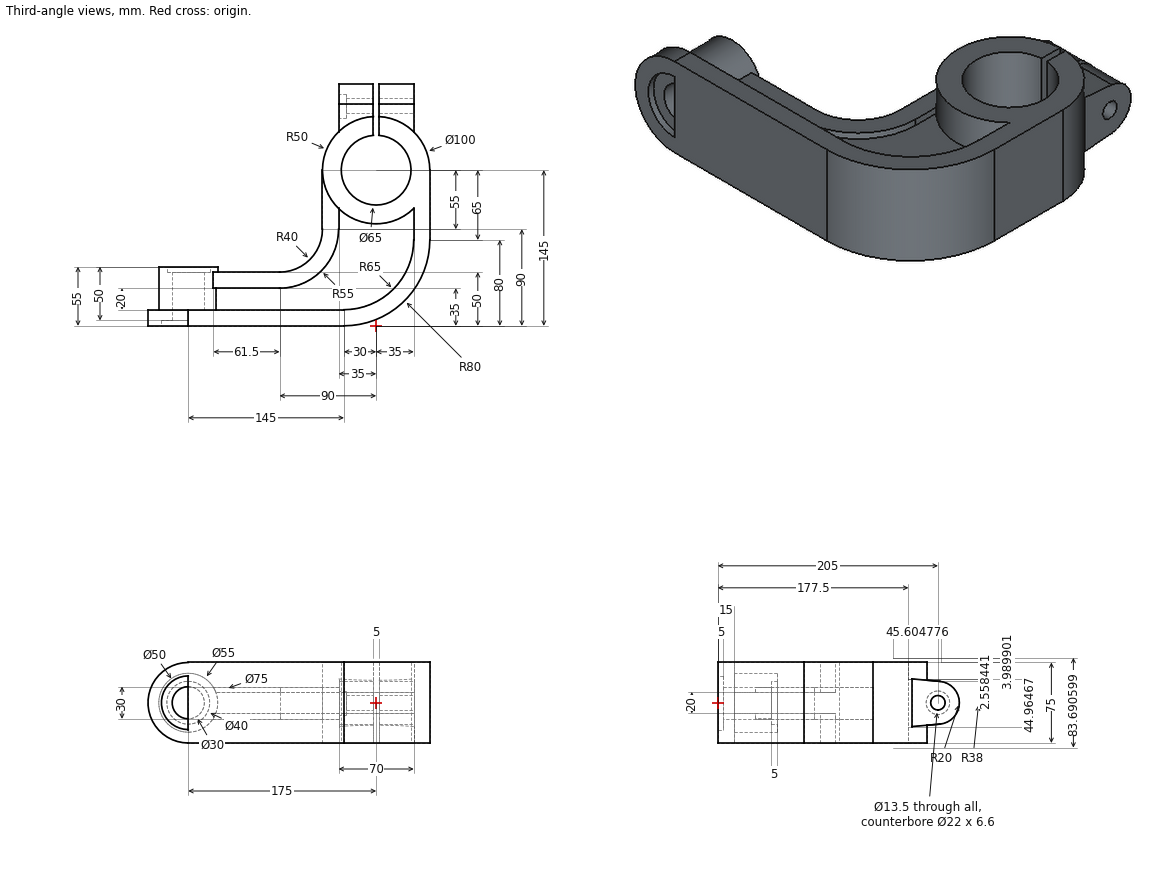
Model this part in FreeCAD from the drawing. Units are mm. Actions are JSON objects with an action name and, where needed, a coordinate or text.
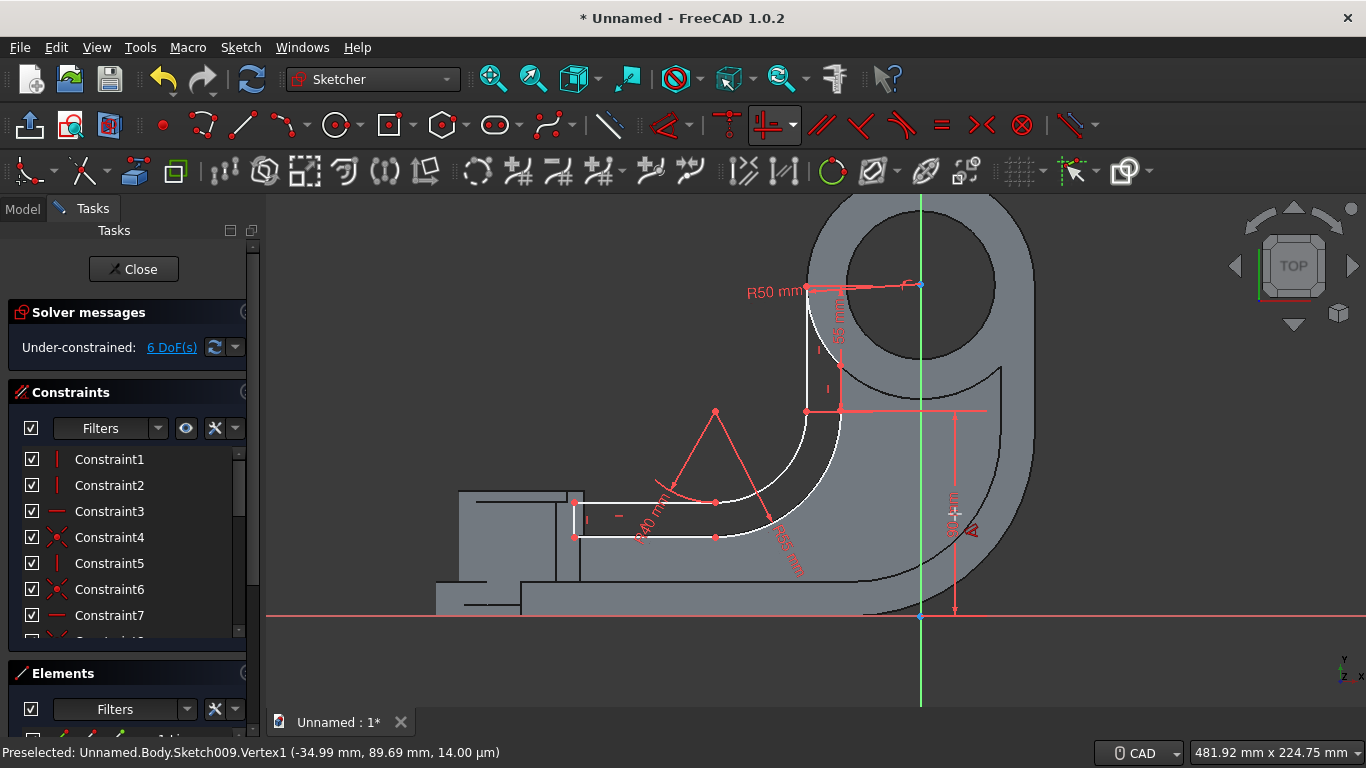
{"action": "left_click", "coordinate": [807, 412]}
{"action": "left_click", "coordinate": [955, 467]}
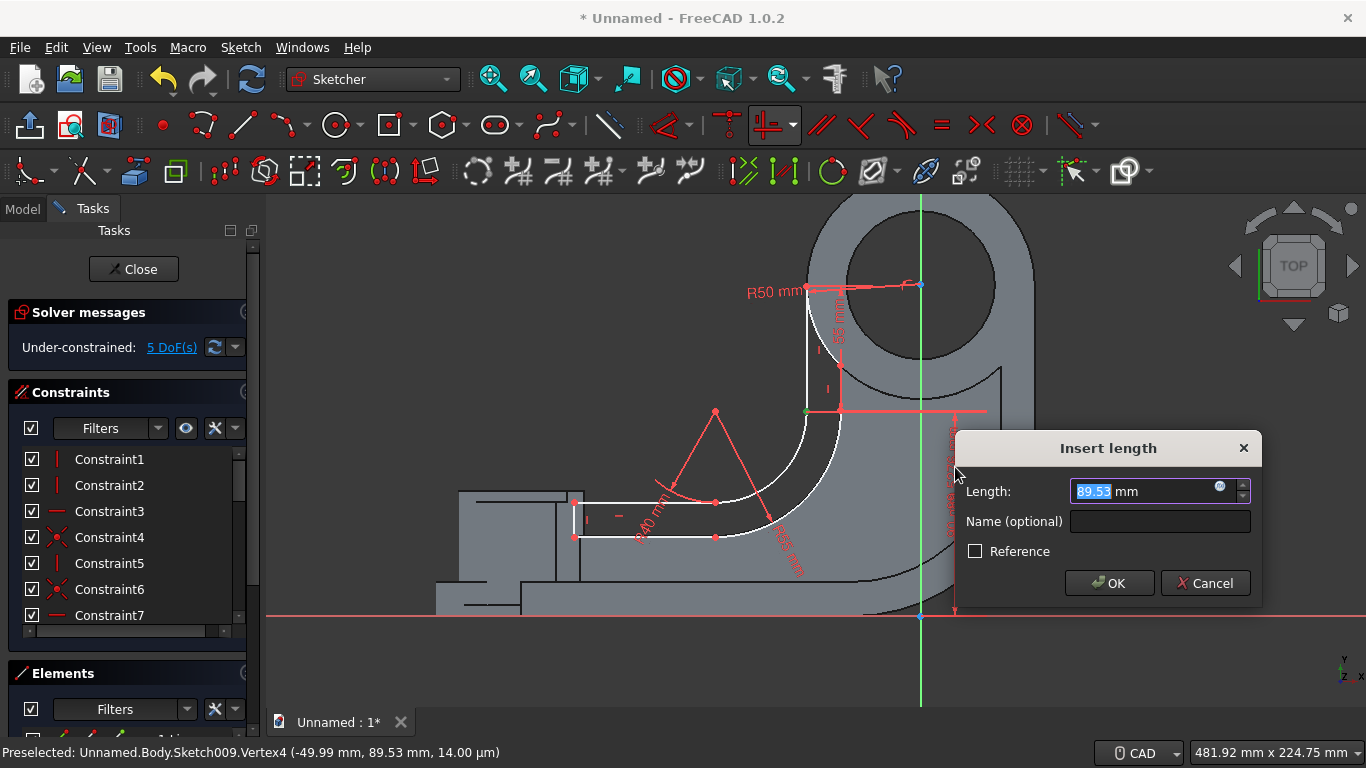
{"action": "type", "text": "90"}
{"action": "key", "text": "Return"}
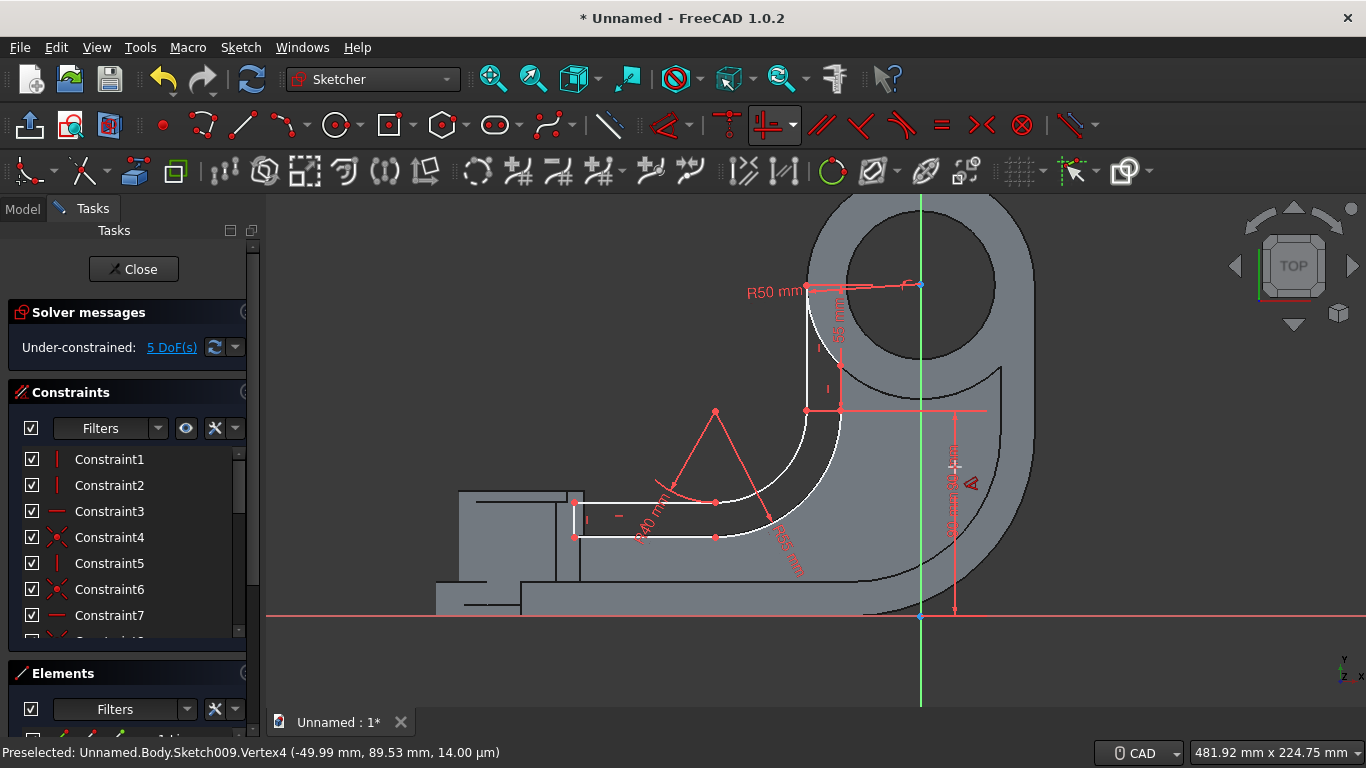
{"action": "left_click", "coordinate": [715, 503]}
{"action": "left_click", "coordinate": [818, 650]}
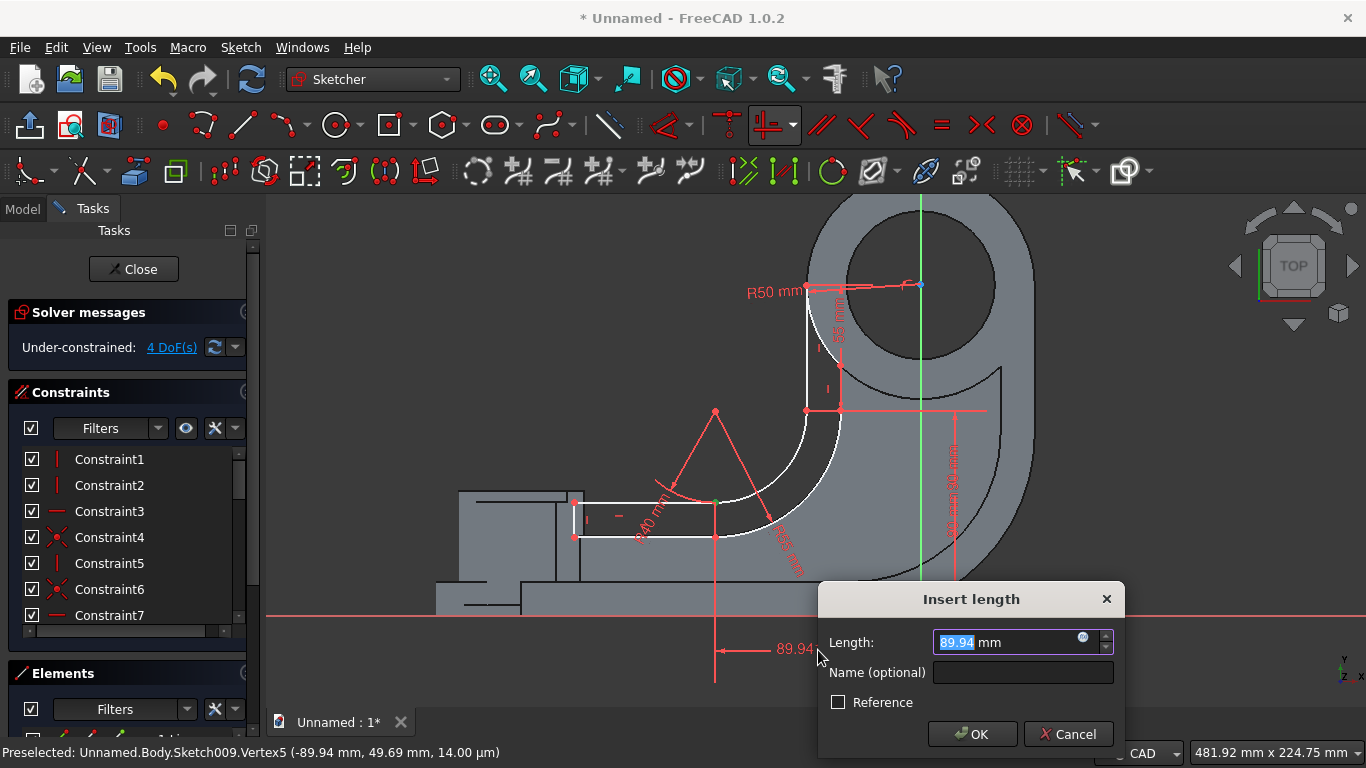
{"action": "type", "text": "90"}
{"action": "key", "text": "Return"}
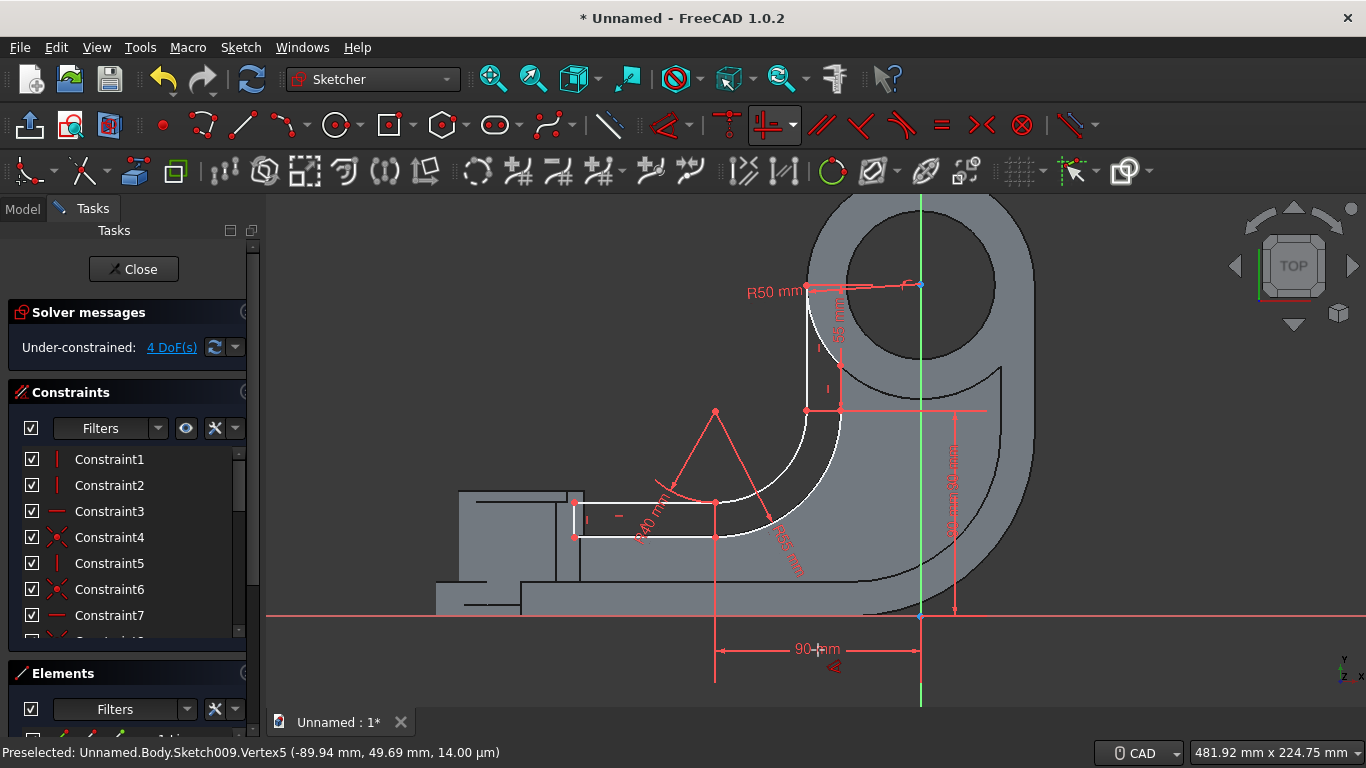
{"action": "left_click", "coordinate": [715, 503]}
{"action": "left_click", "coordinate": [955, 559]}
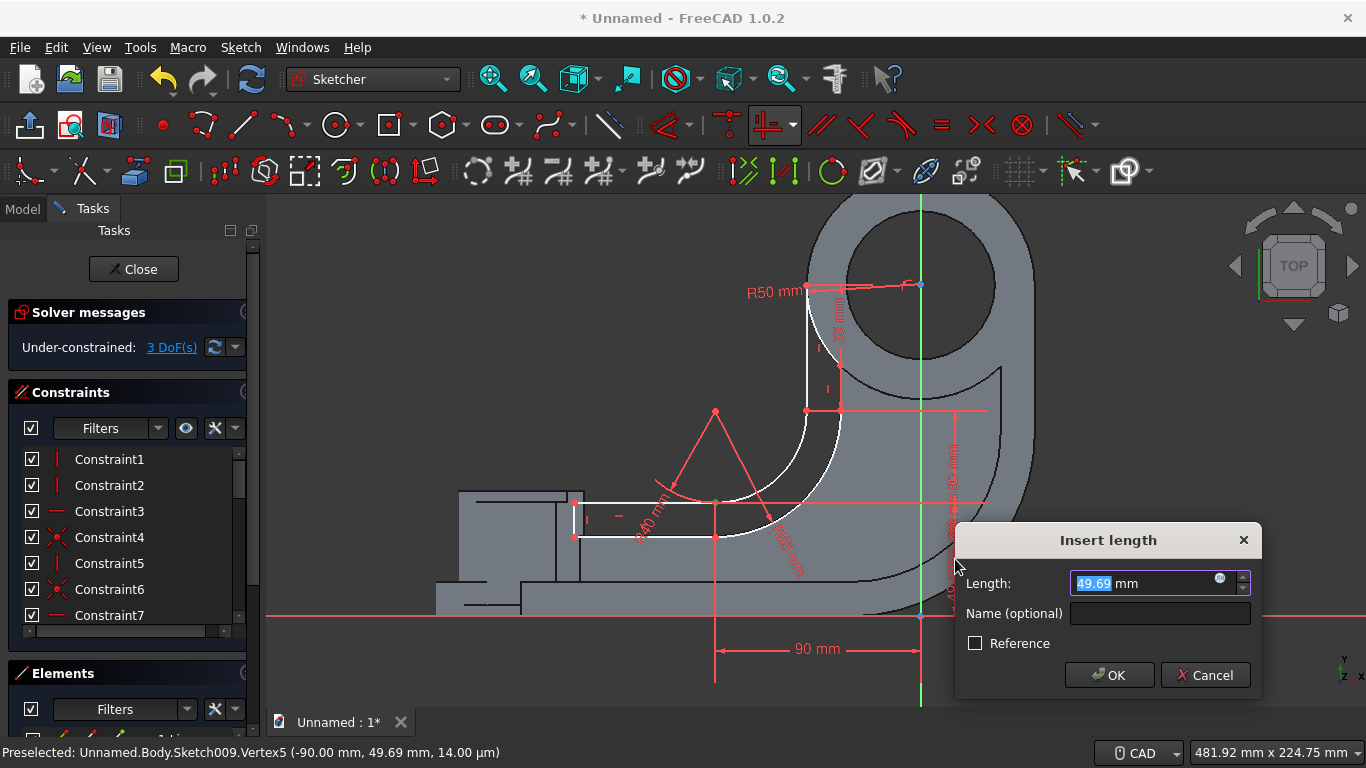
{"action": "type", "text": "50"}
{"action": "key", "text": "Return"}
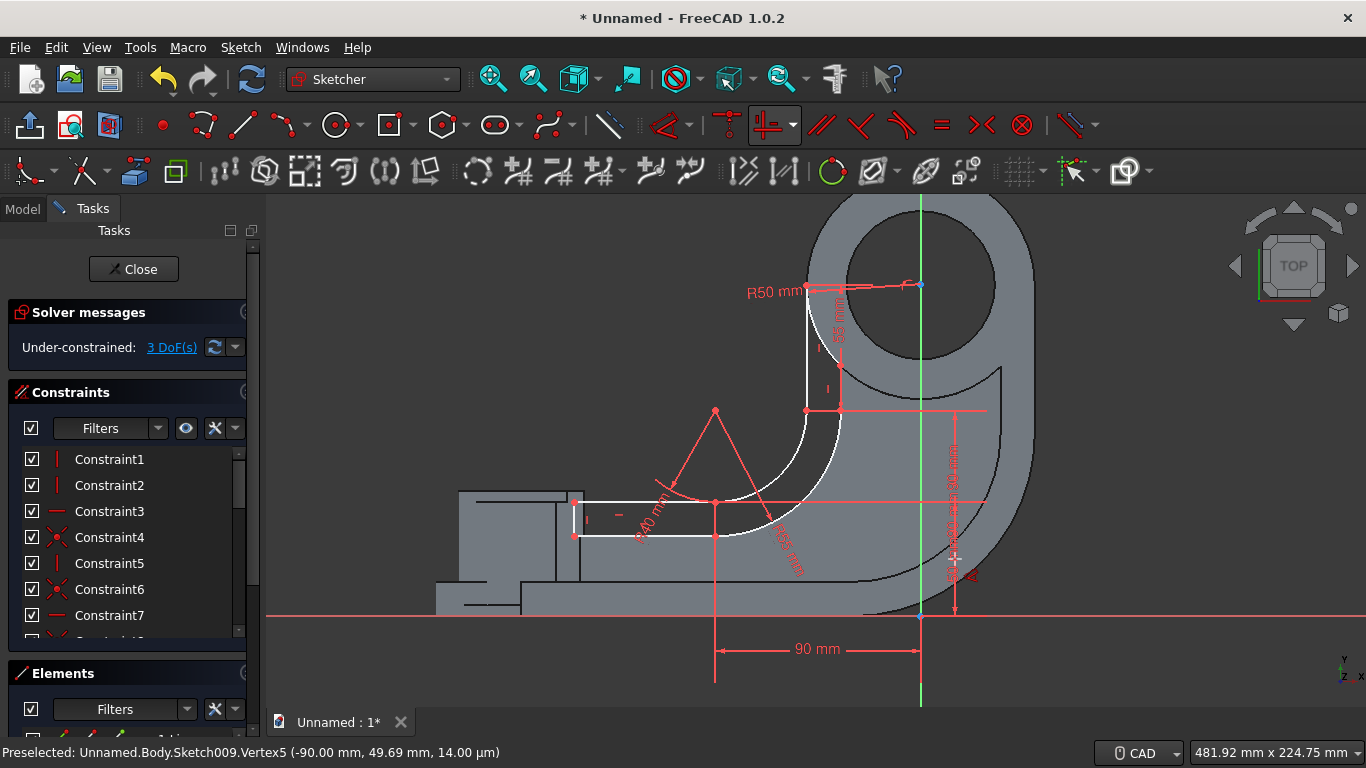
{"action": "left_click", "coordinate": [715, 536]}
{"action": "left_click", "coordinate": [746, 650]}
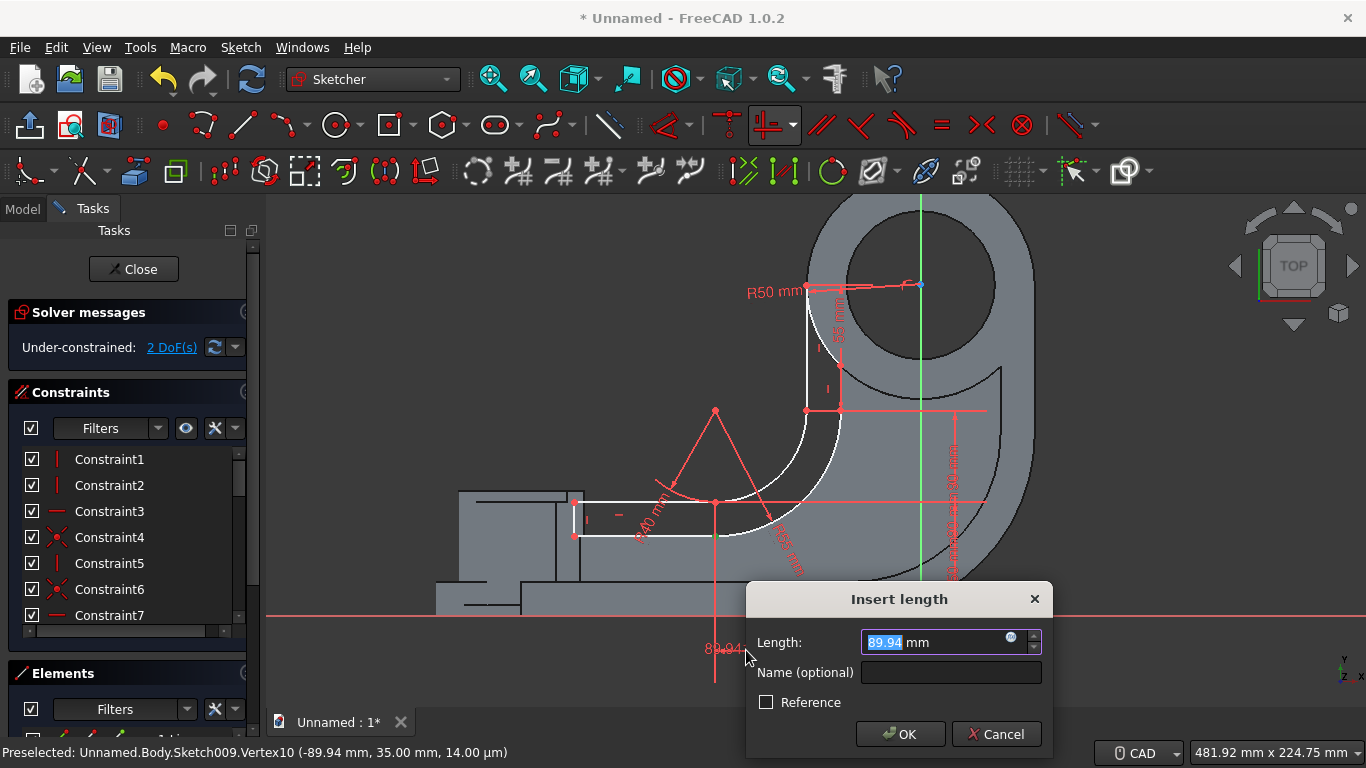
{"action": "type", "text": "90"}
{"action": "key", "text": "Return"}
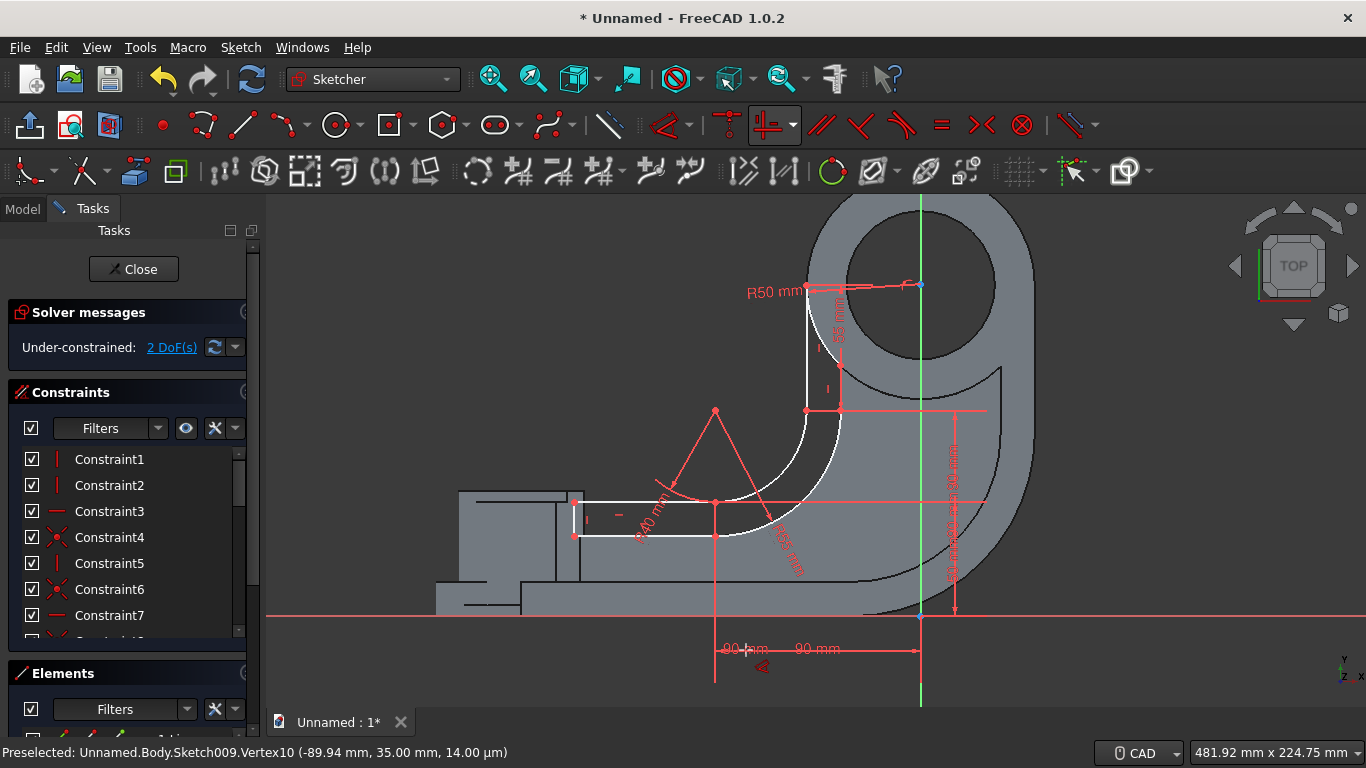
{"action": "left_click", "coordinate": [673, 502]}
{"action": "left_click", "coordinate": [645, 468]}